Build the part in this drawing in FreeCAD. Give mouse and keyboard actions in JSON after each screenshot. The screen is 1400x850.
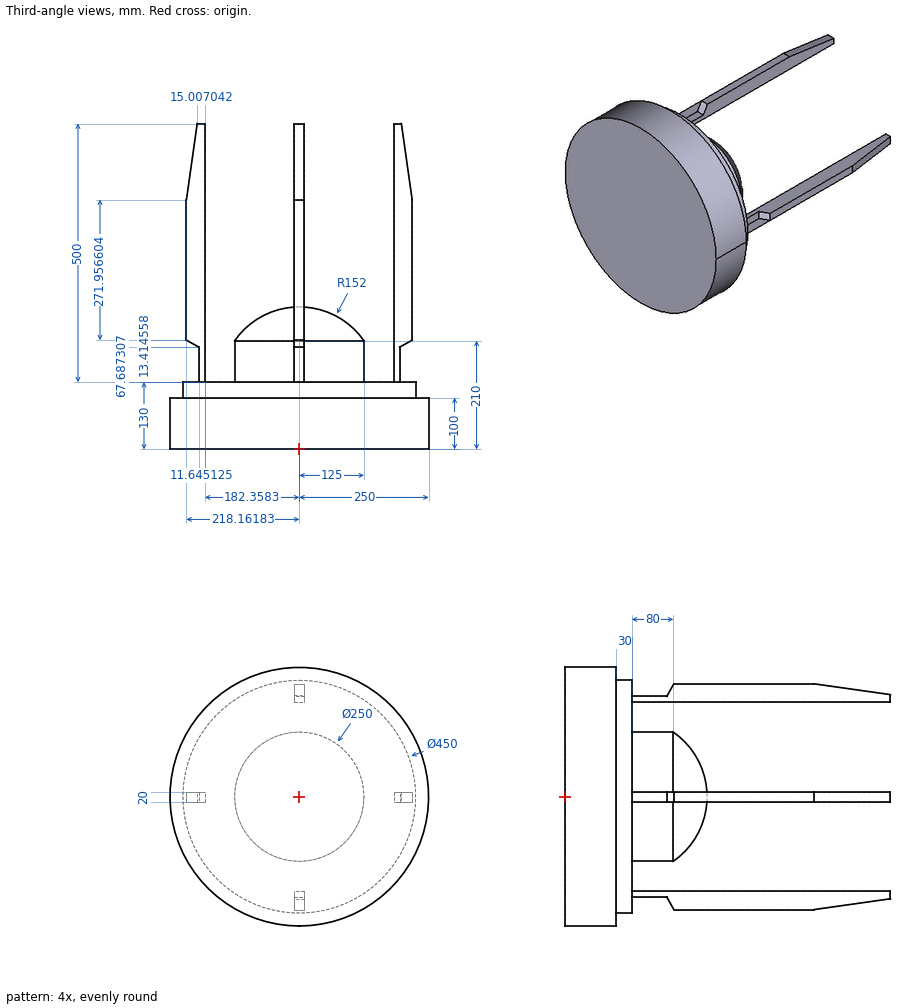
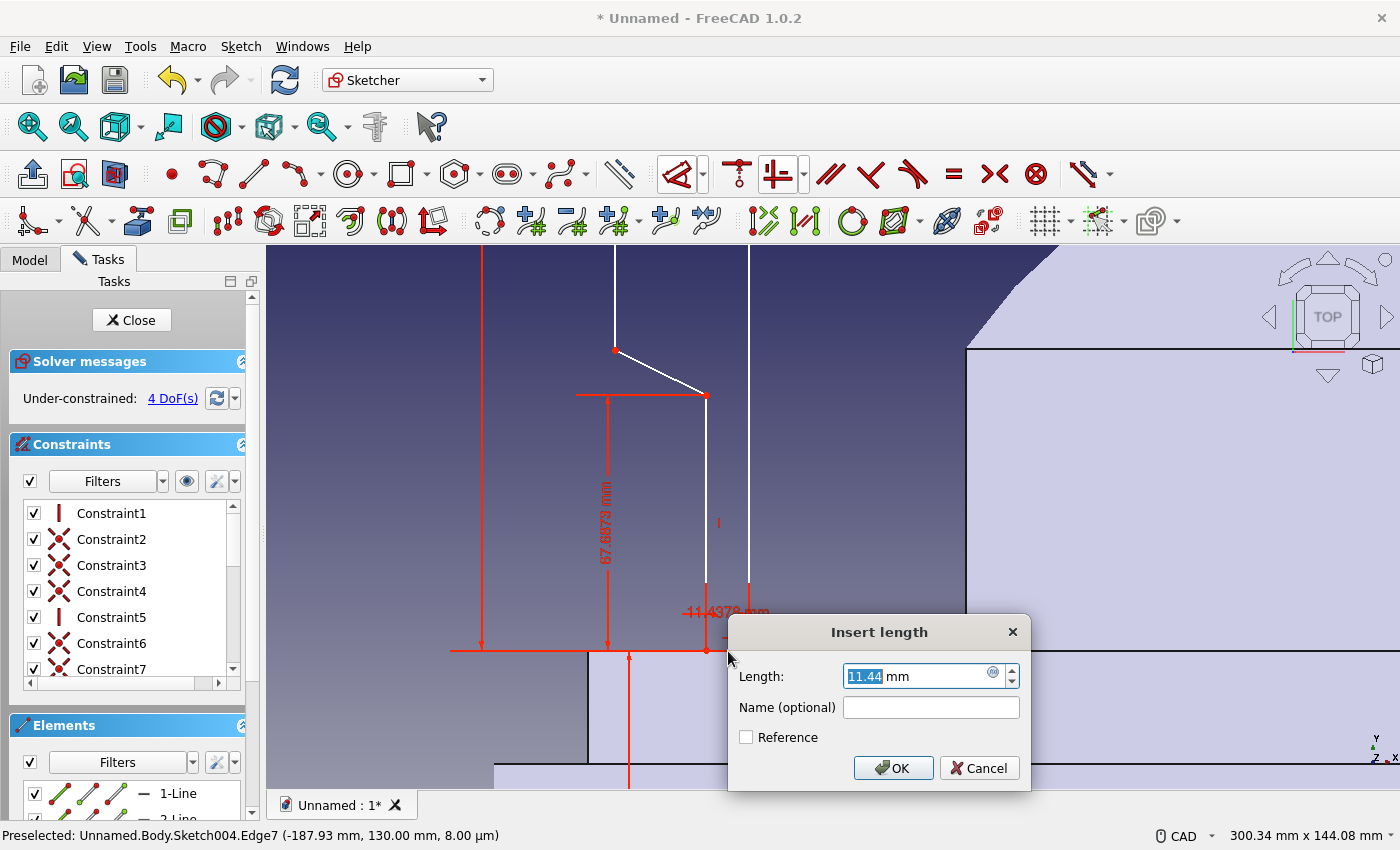
{"action": "type", "text": "11.645125"}
{"action": "key", "text": "Return"}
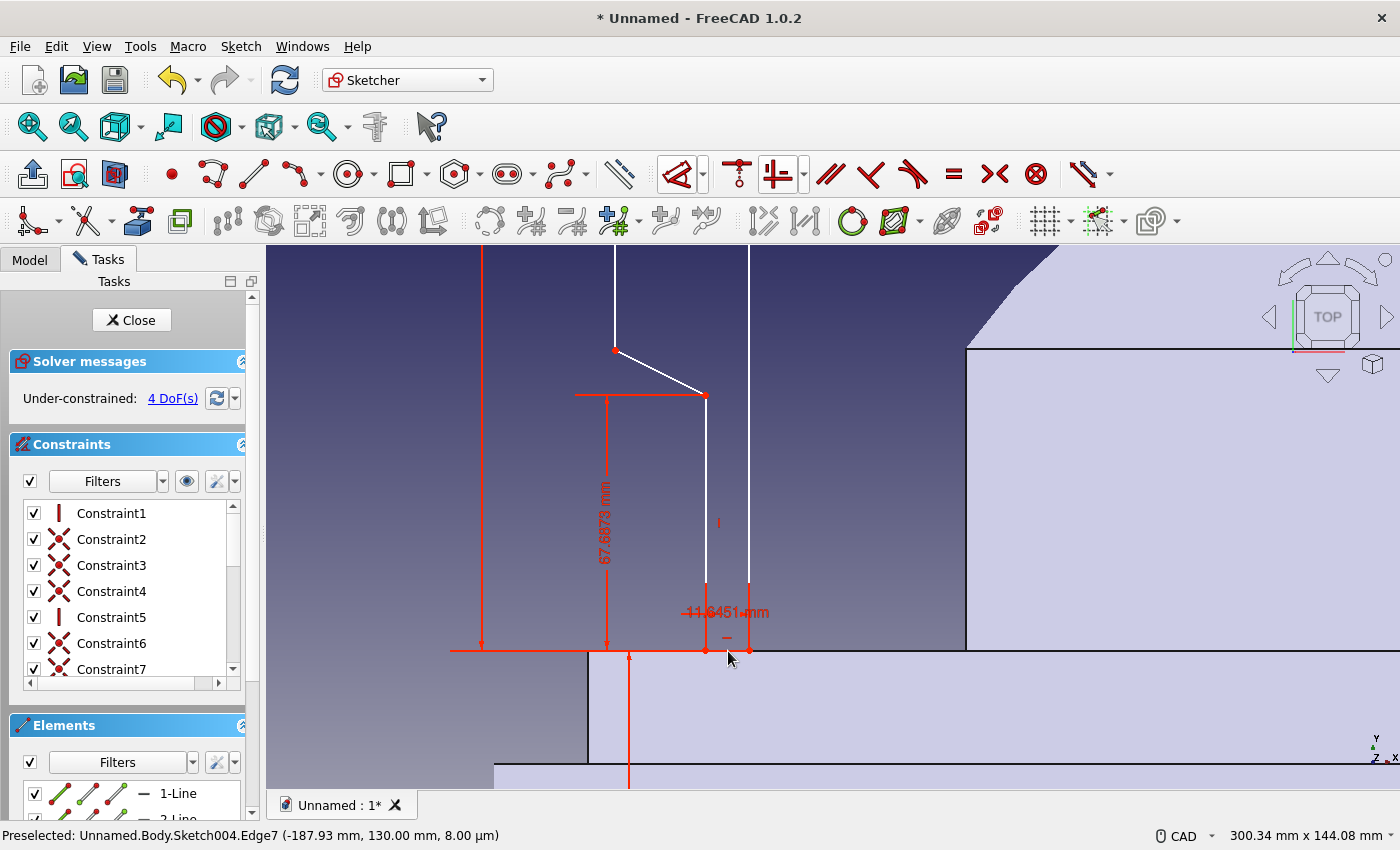
{"action": "scroll", "coordinate": [724, 605], "scroll_direction": "down", "scroll_amount": 10}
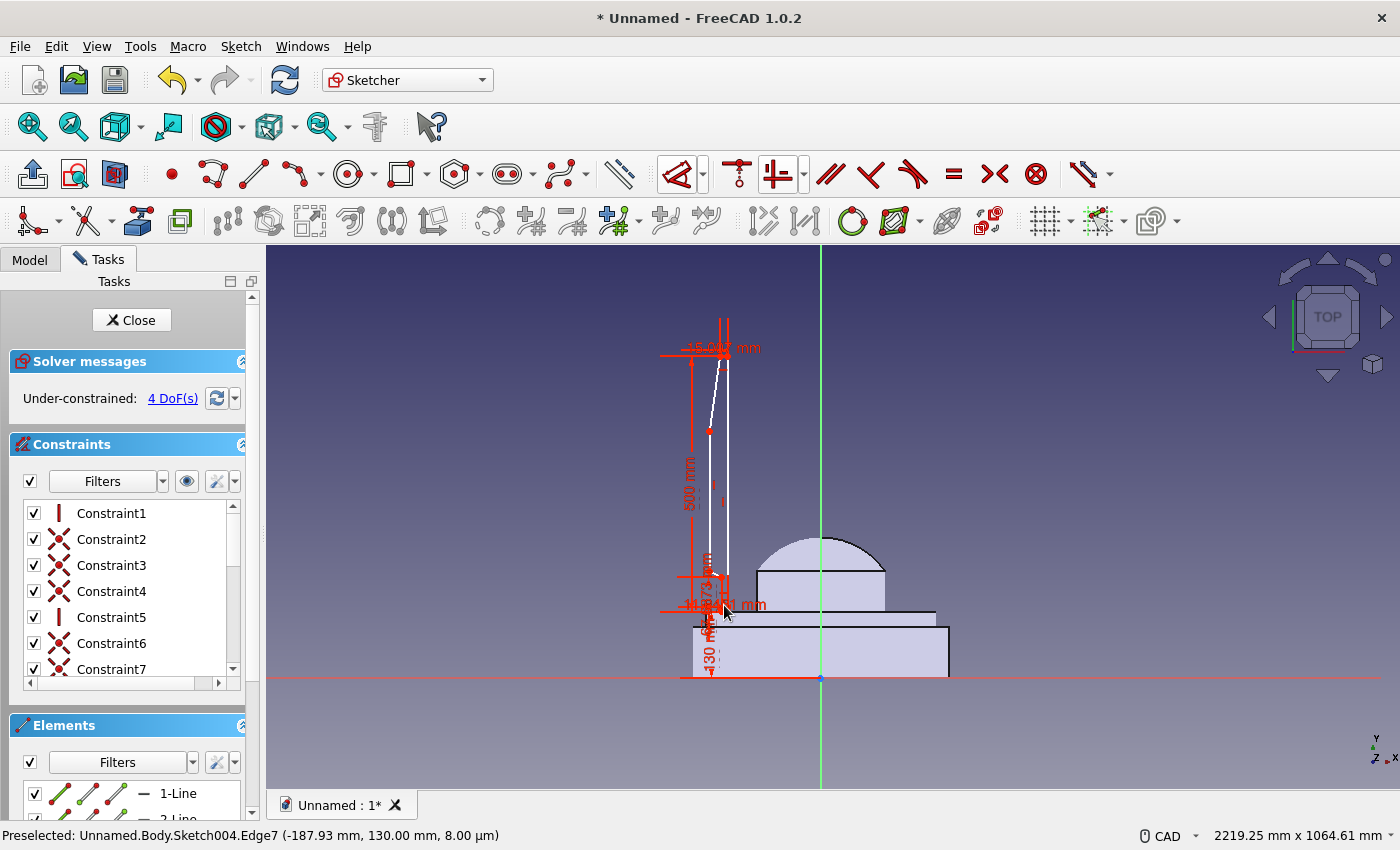
{"action": "scroll", "coordinate": [728, 612], "scroll_direction": "up", "scroll_amount": 4}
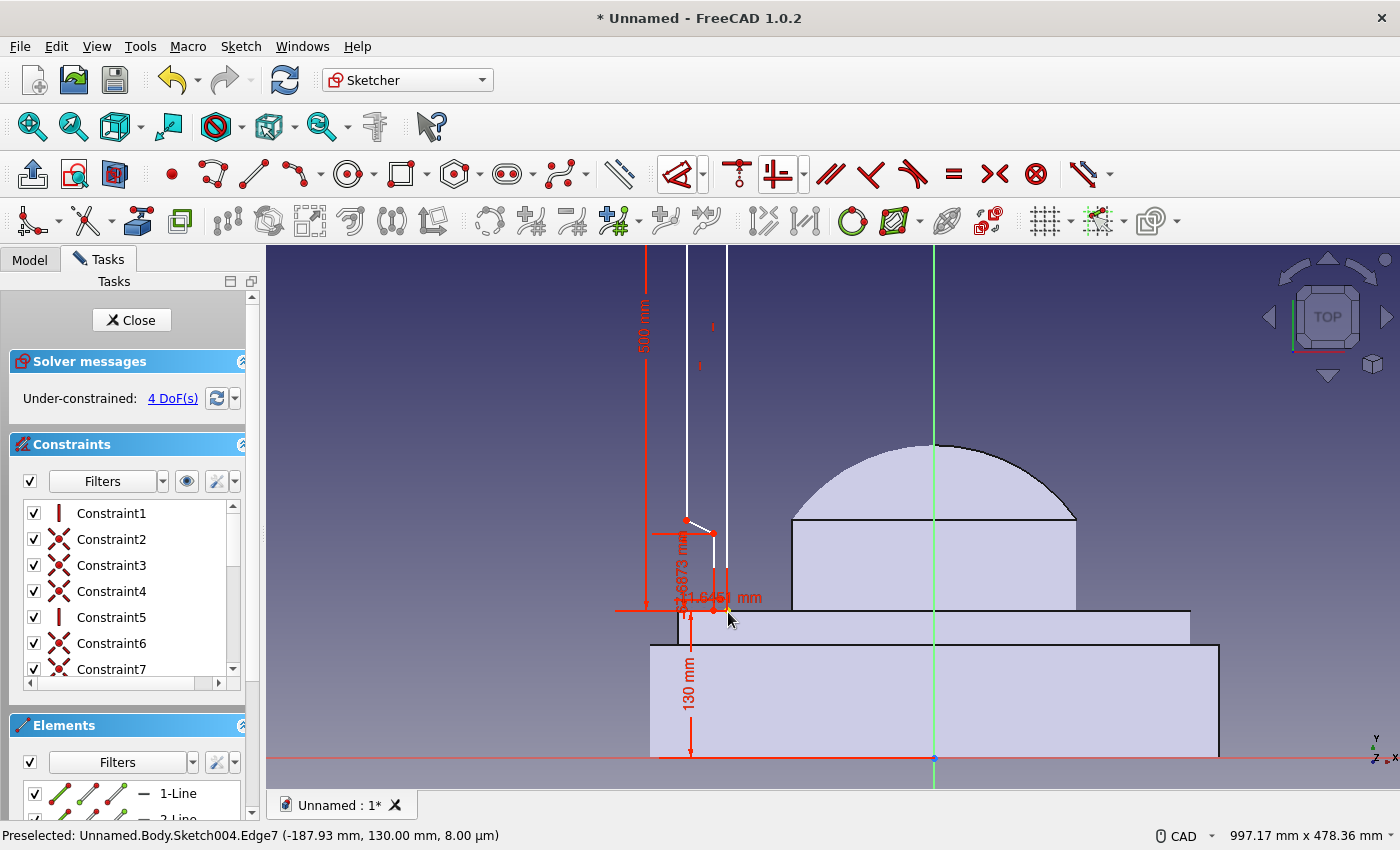
{"action": "left_click", "coordinate": [727, 611]}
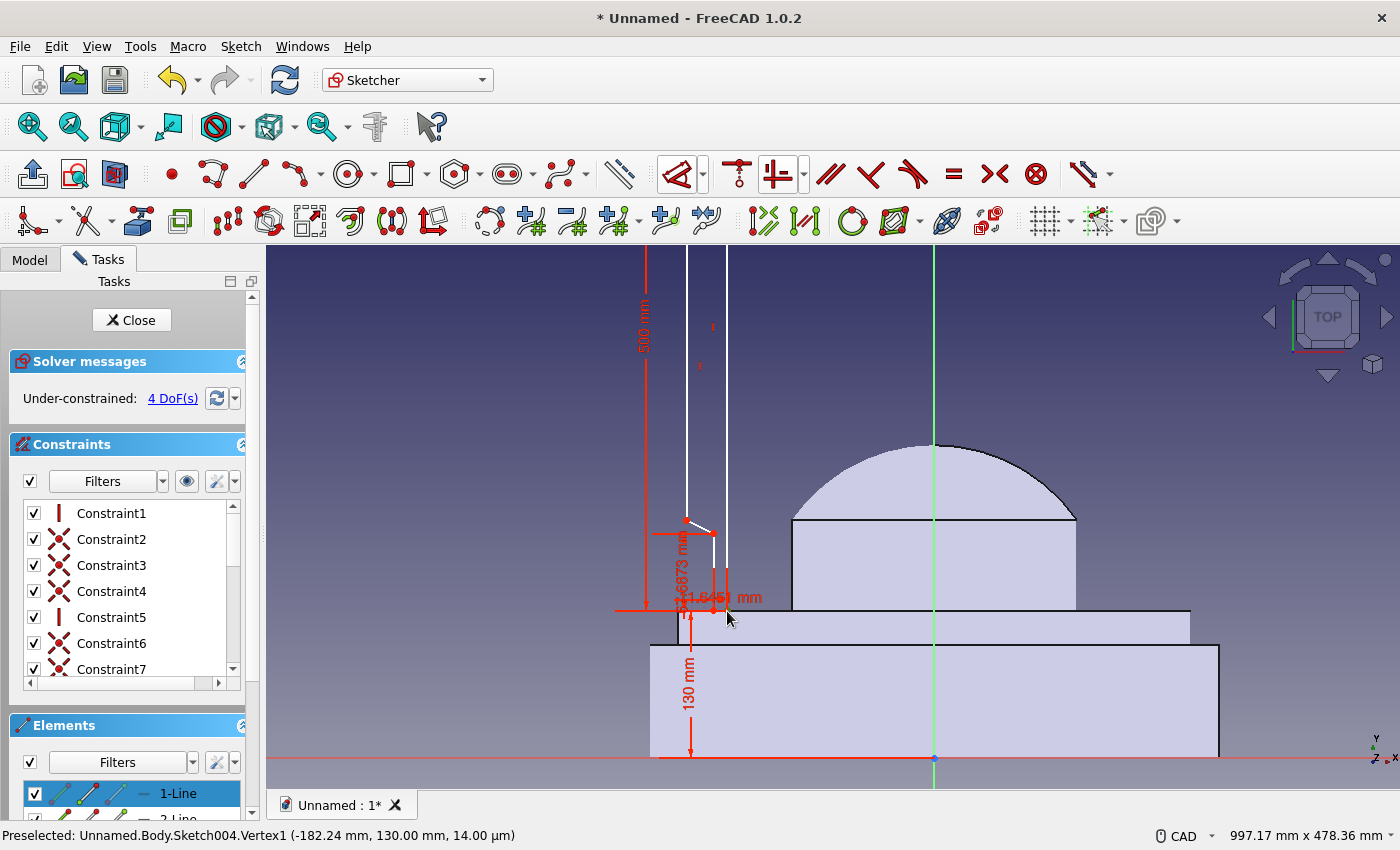
{"action": "left_click", "coordinate": [702, 174]}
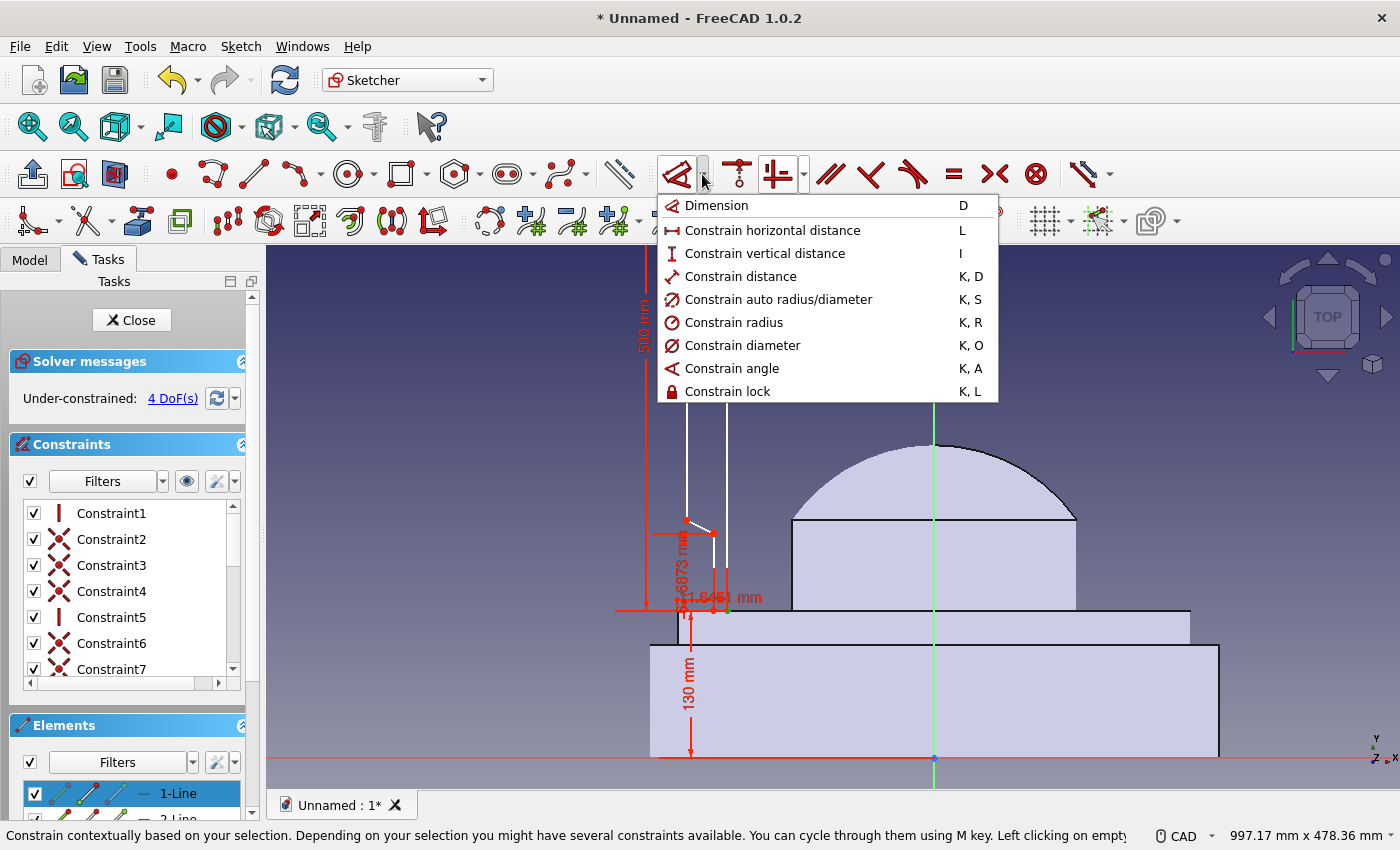
{"action": "left_click", "coordinate": [828, 230]}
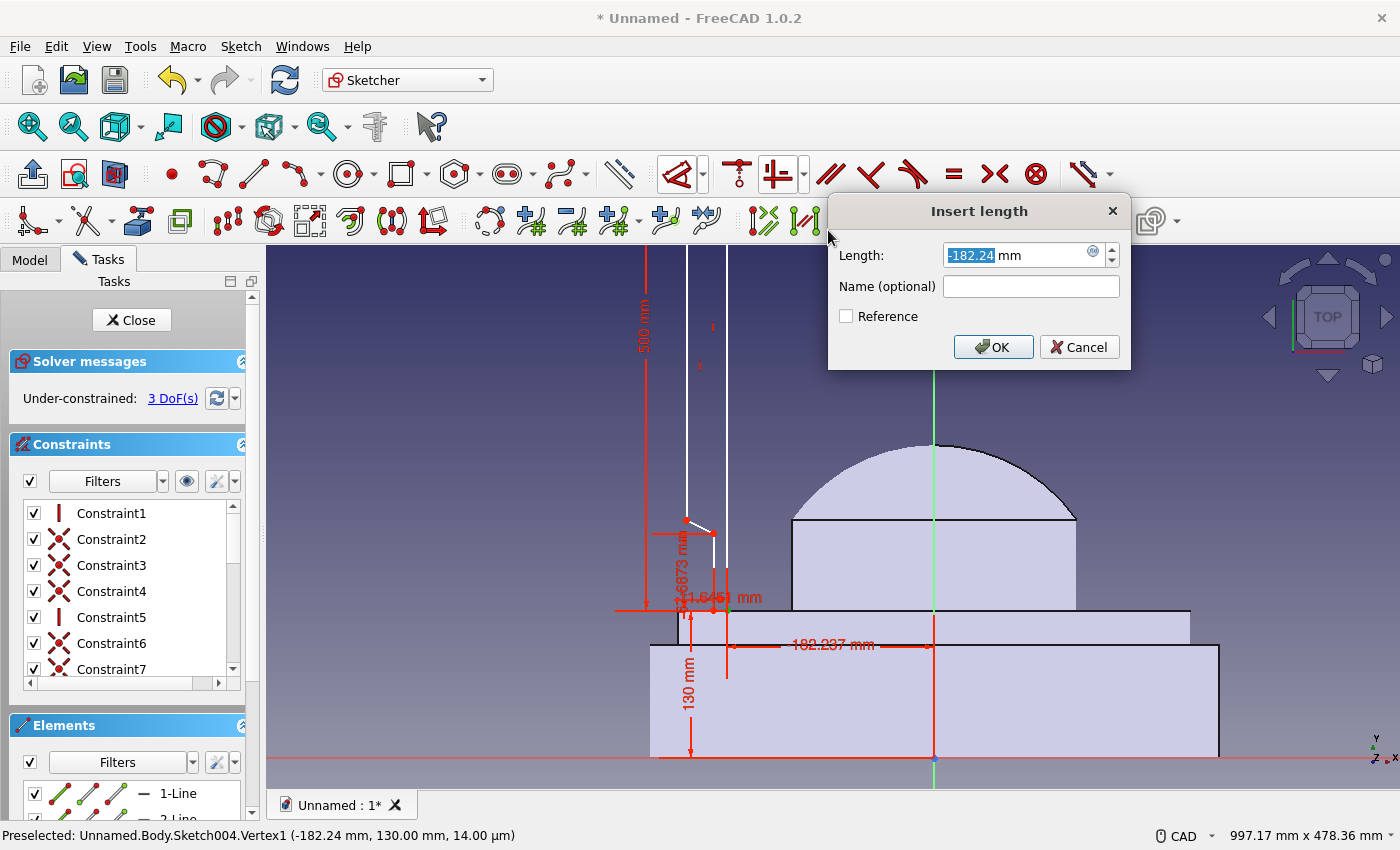
{"action": "type", "text": "-182.3583"}
{"action": "key", "text": "Return"}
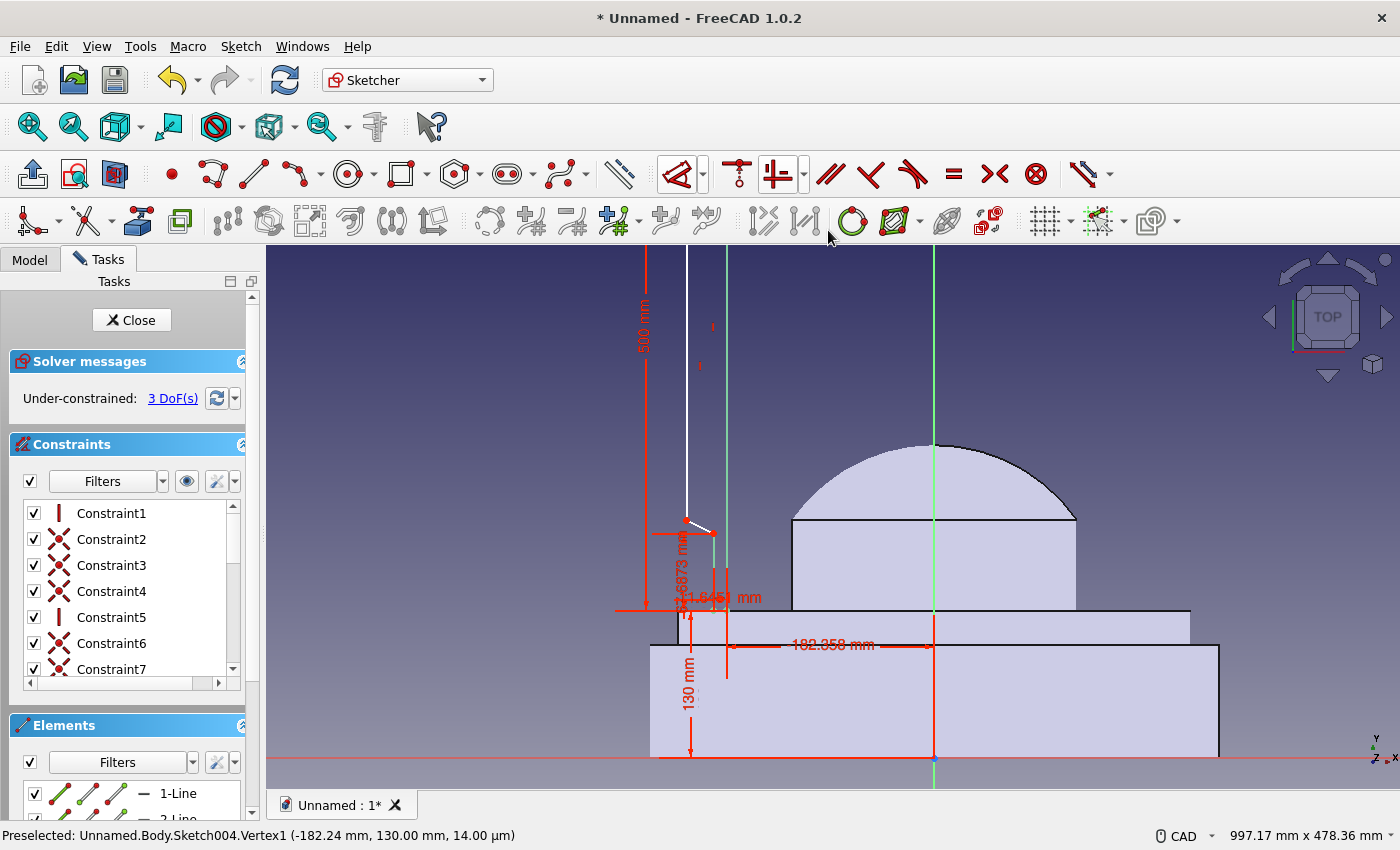
{"action": "left_click", "coordinate": [687, 303]}